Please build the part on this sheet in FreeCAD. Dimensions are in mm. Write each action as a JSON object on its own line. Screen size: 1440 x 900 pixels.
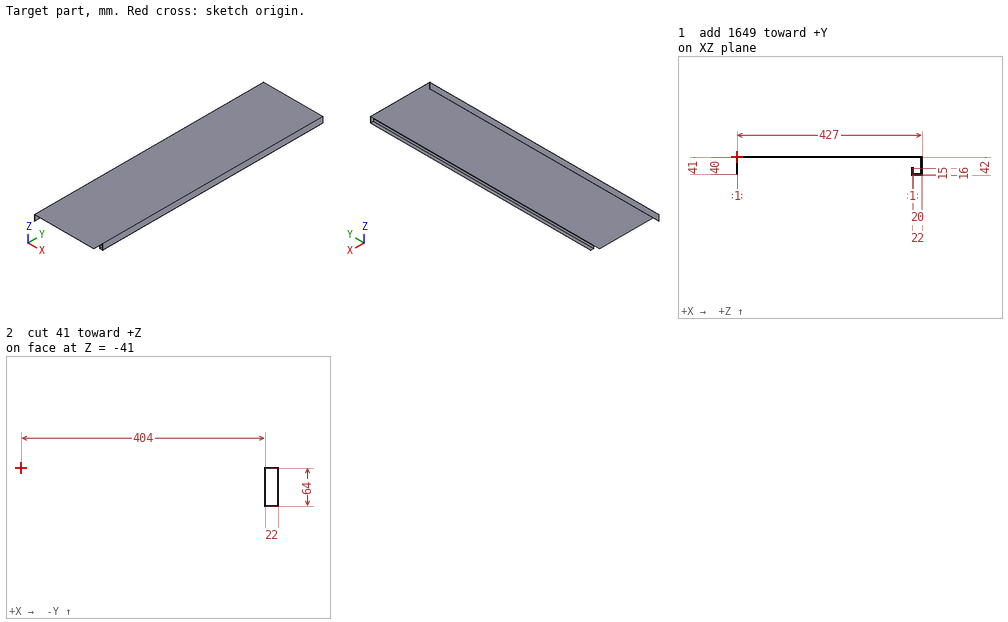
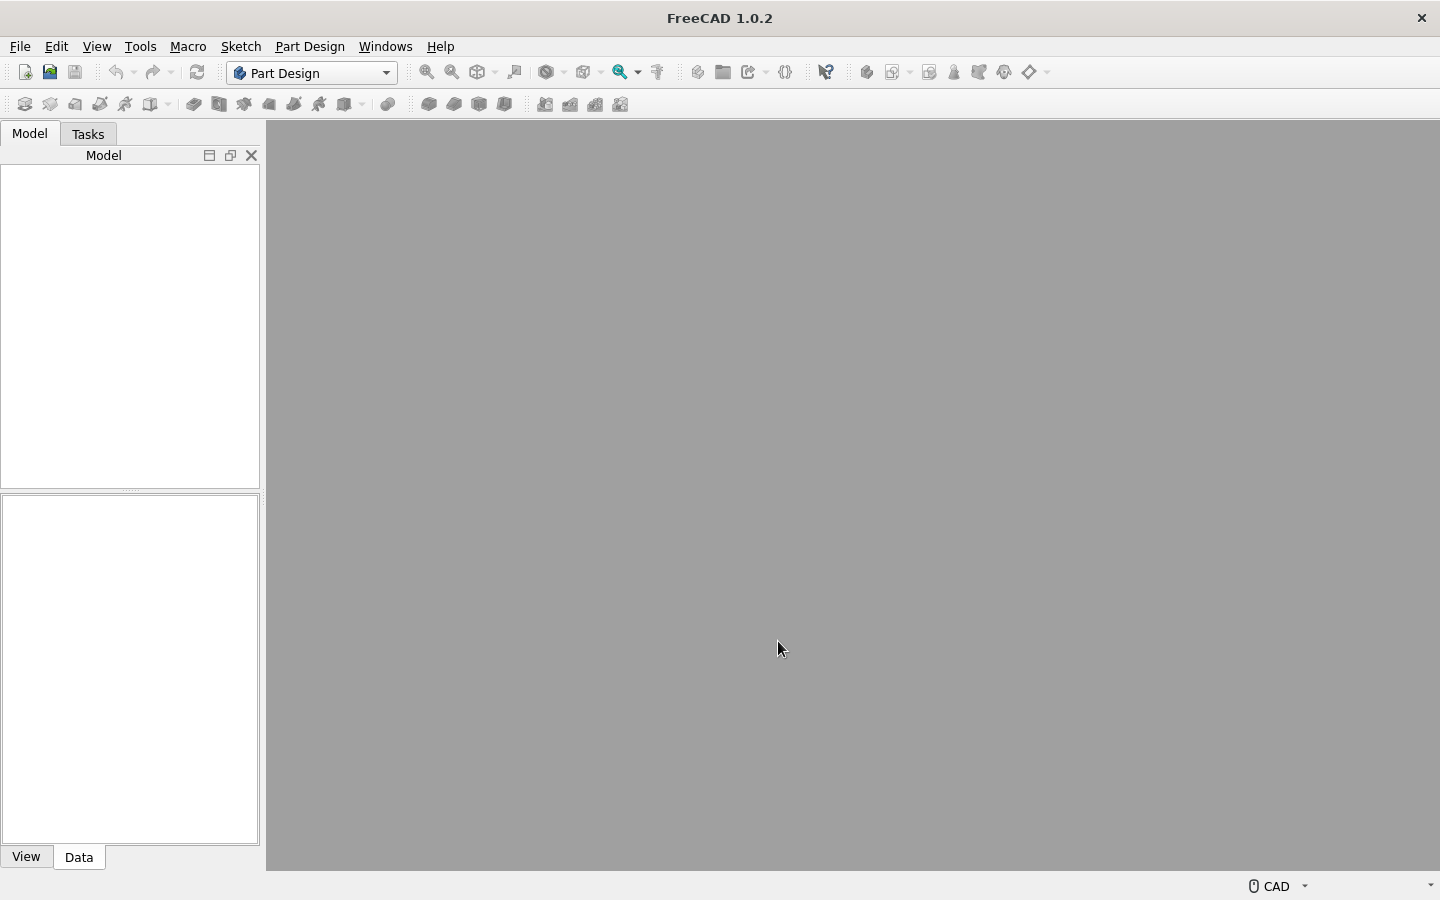
{"action": "left_click", "coordinate": [25, 72]}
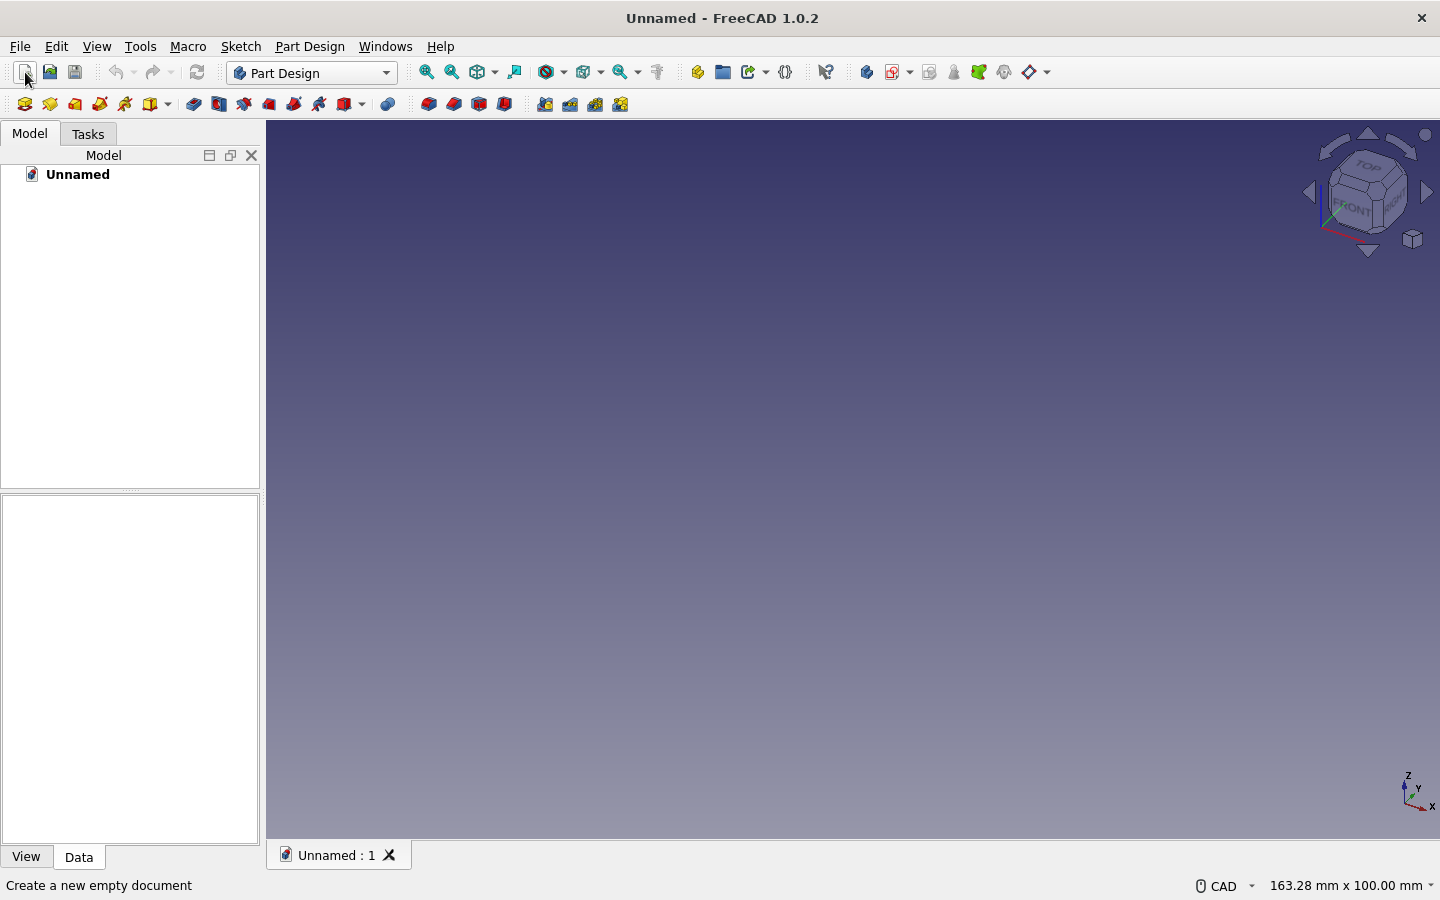
{"action": "left_click", "coordinate": [892, 72]}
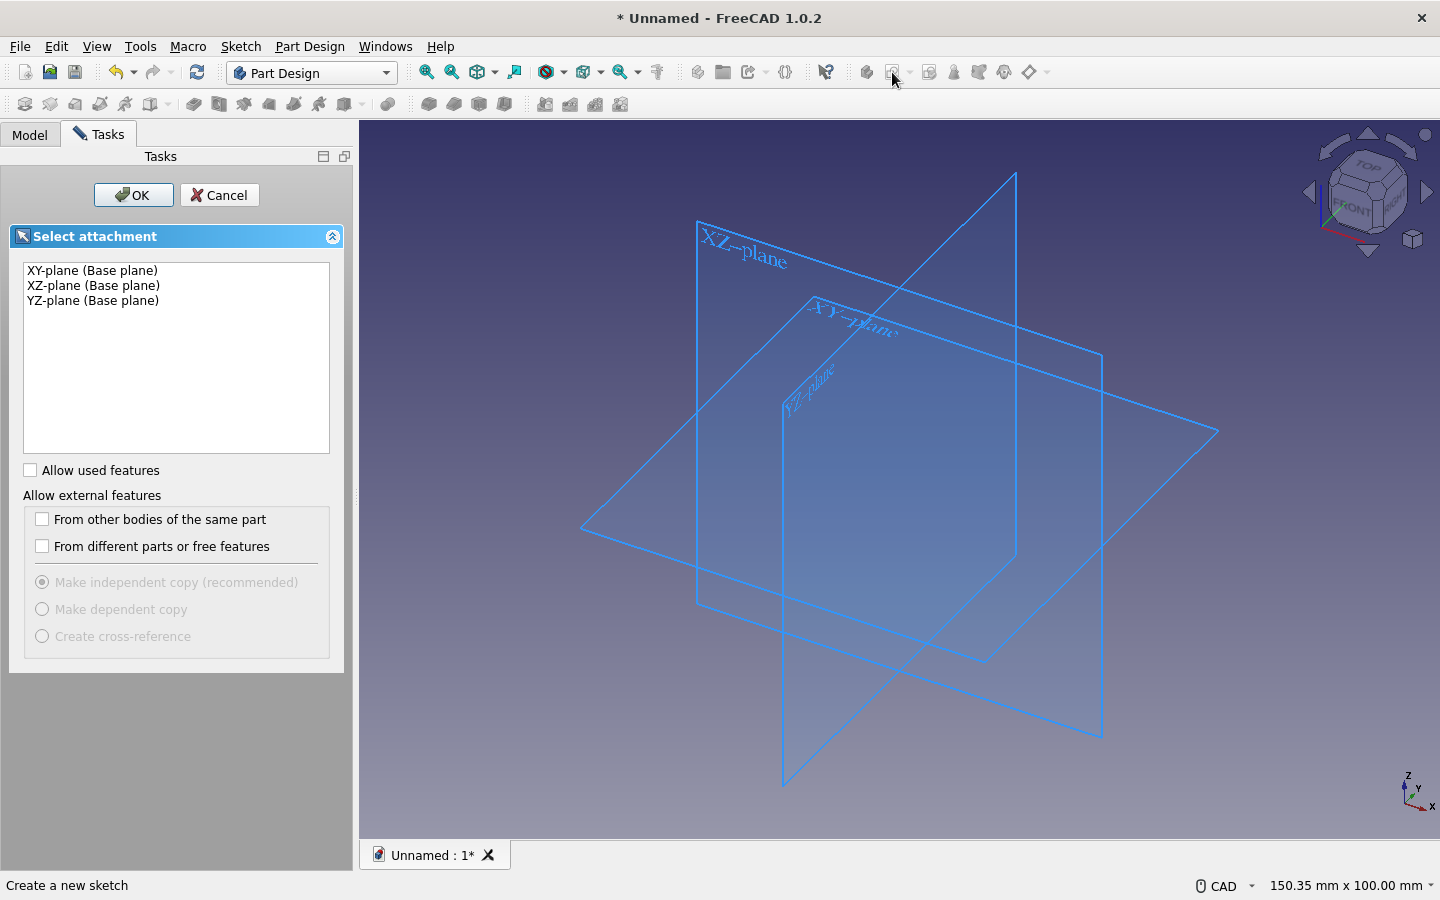
{"action": "left_click", "coordinate": [84, 286]}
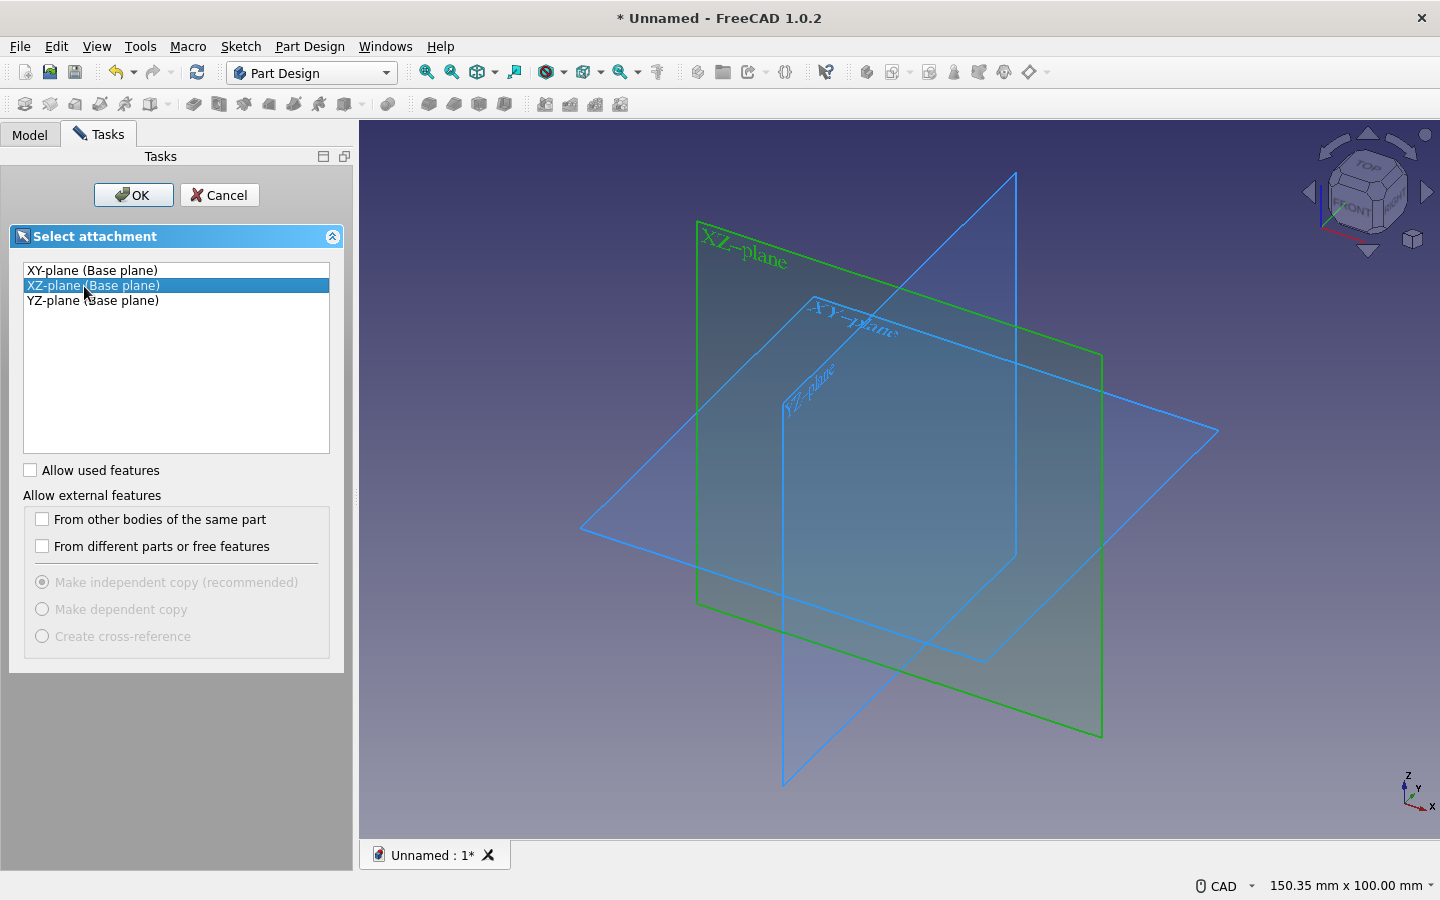
{"action": "left_click", "coordinate": [134, 195]}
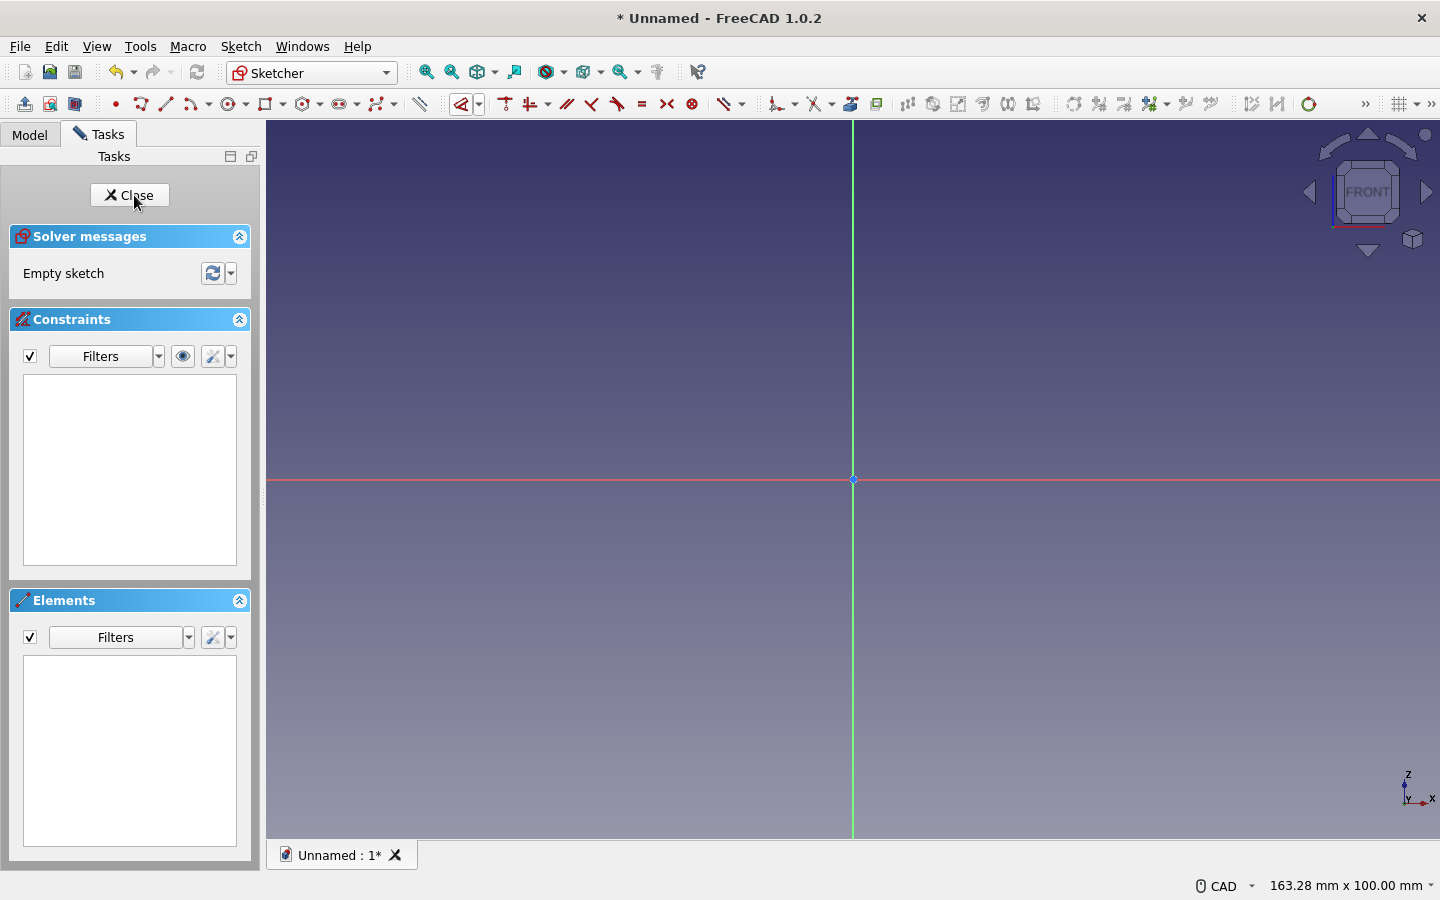
{"action": "scroll", "coordinate": [294, 432], "scroll_direction": "down", "scroll_amount": 7}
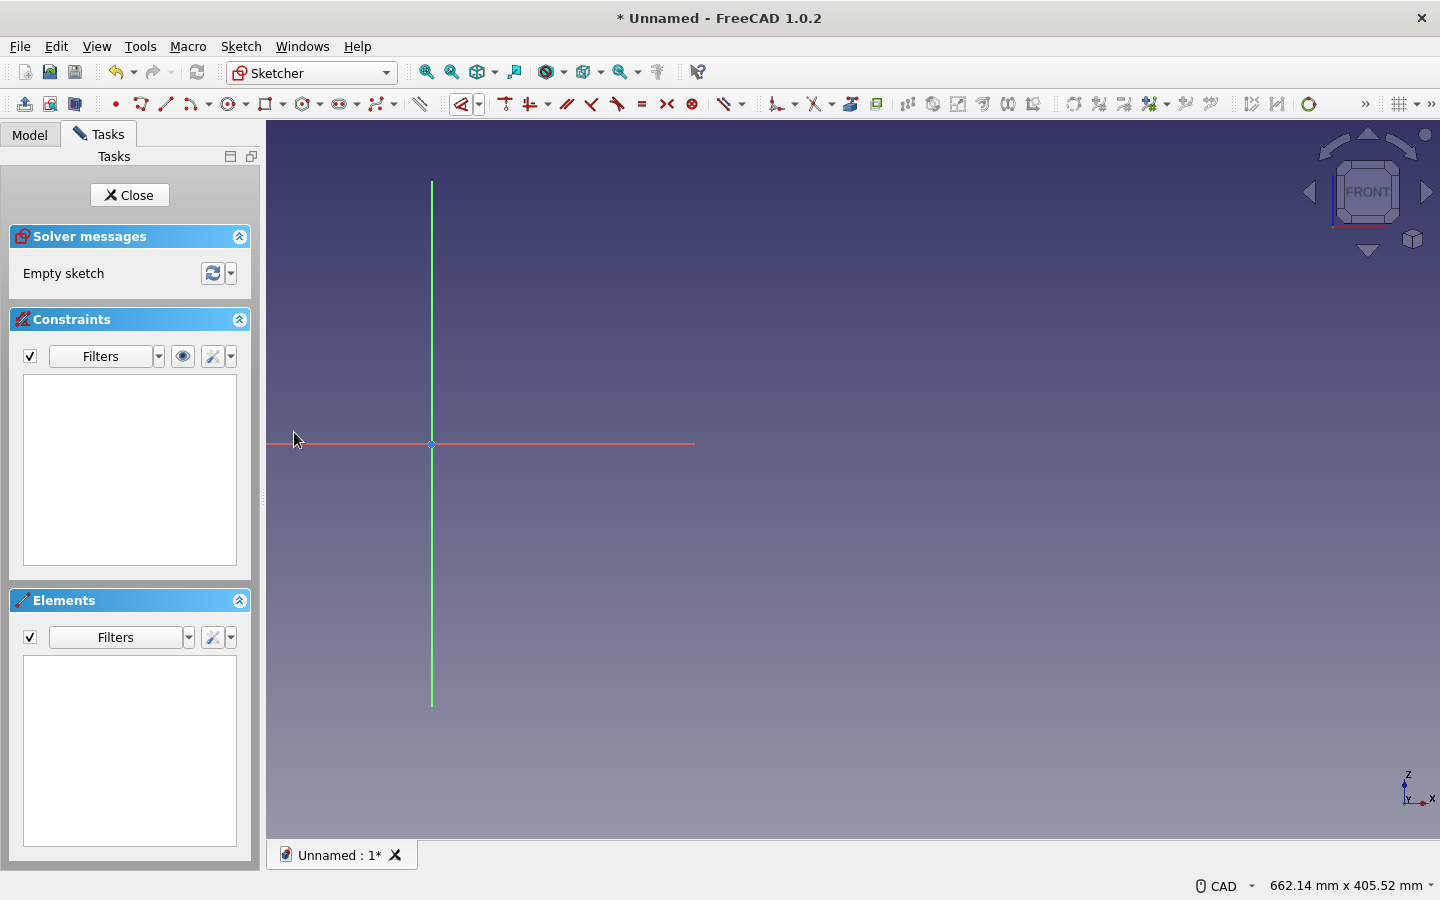
{"action": "left_click", "coordinate": [141, 104]}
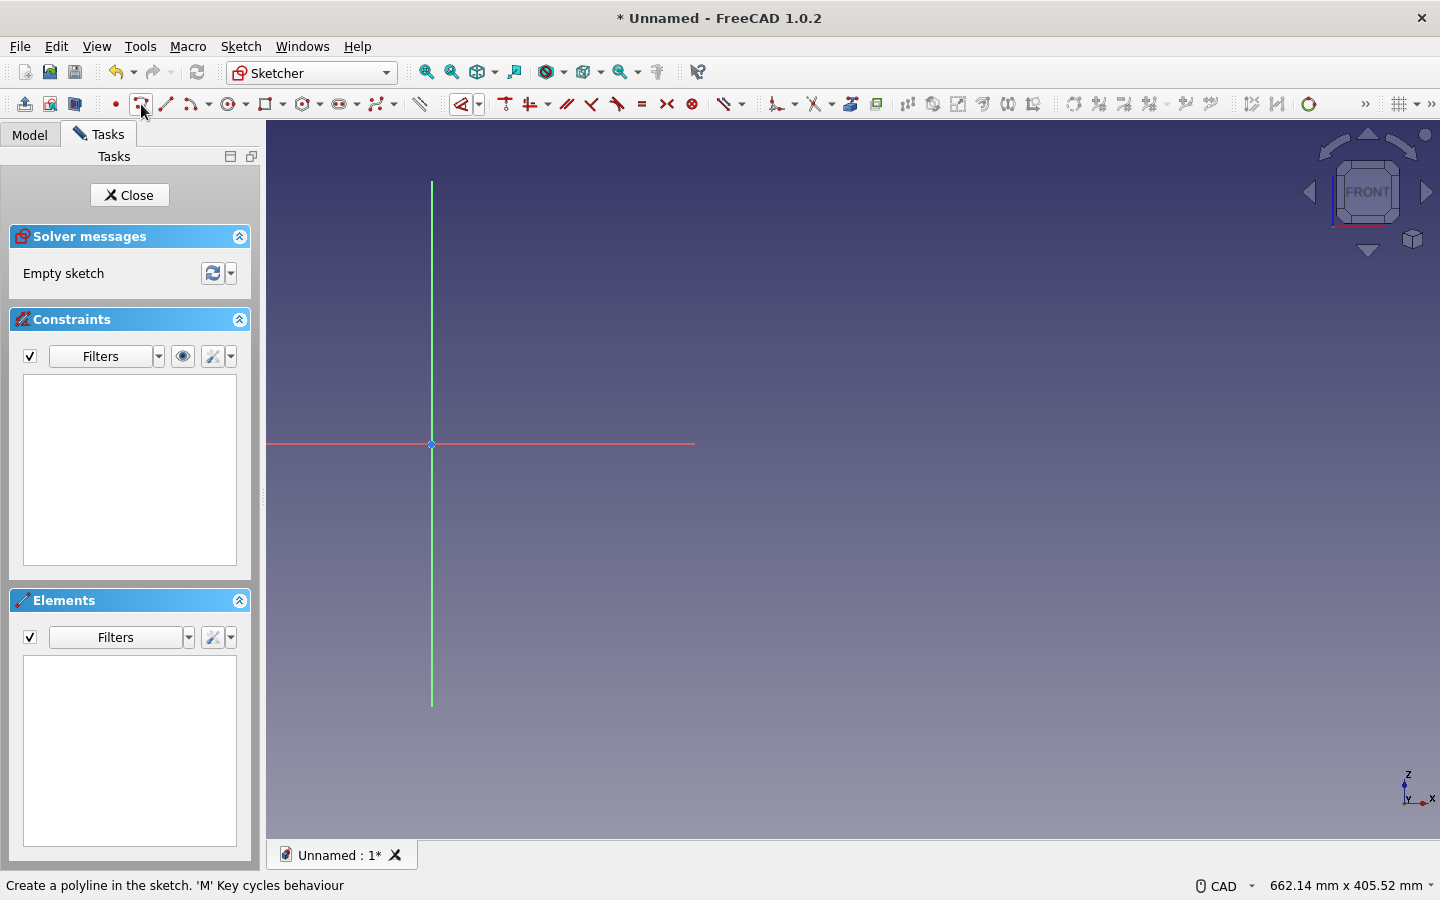
{"action": "left_click", "coordinate": [432, 444]}
{"action": "left_click", "coordinate": [441, 515]}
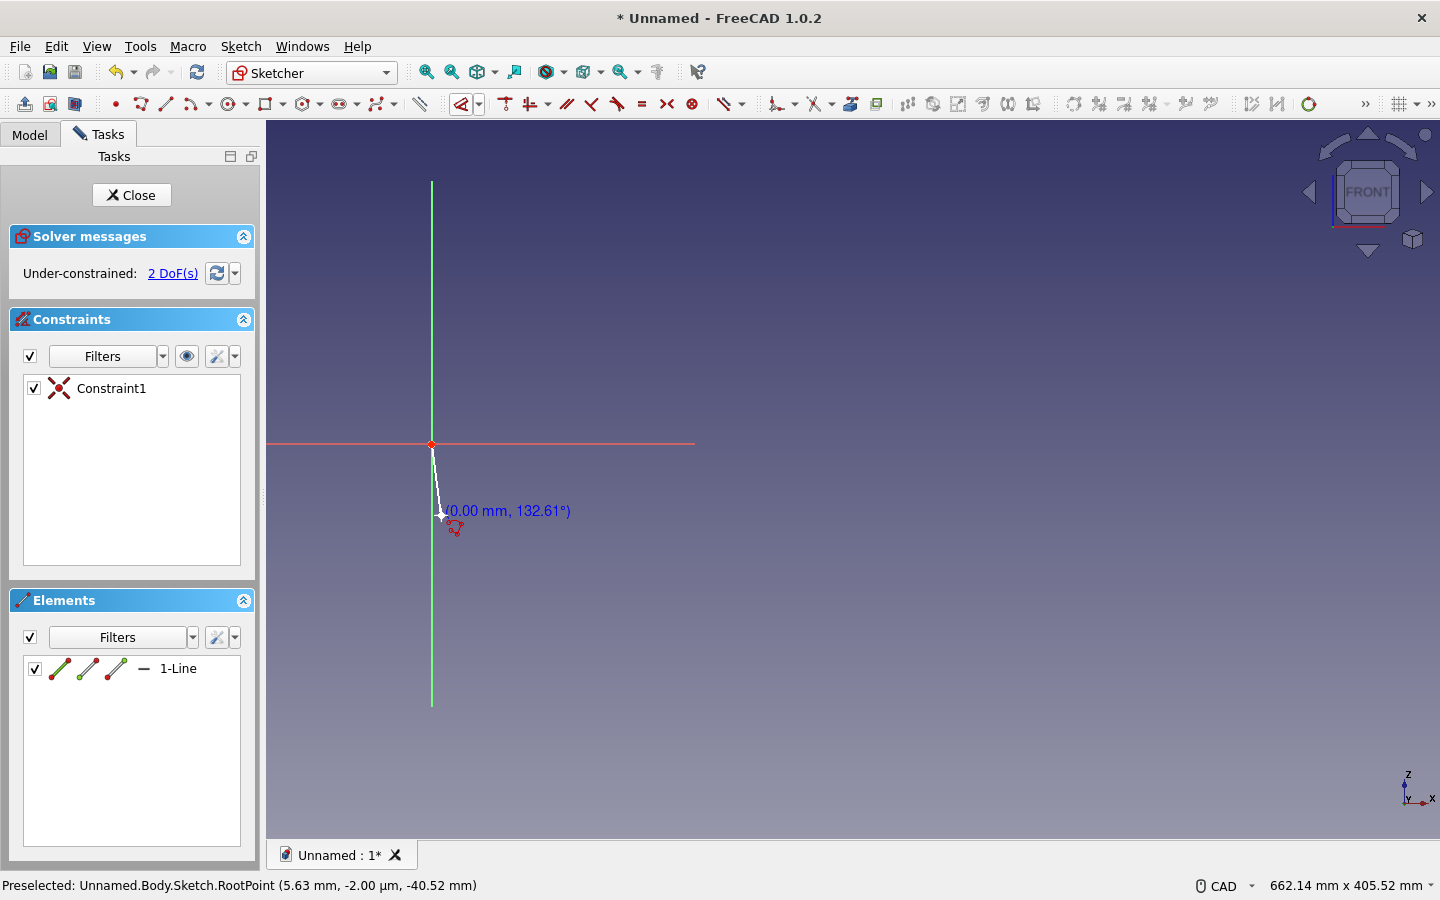
{"action": "scroll", "coordinate": [430, 515], "scroll_direction": "up", "scroll_amount": 11}